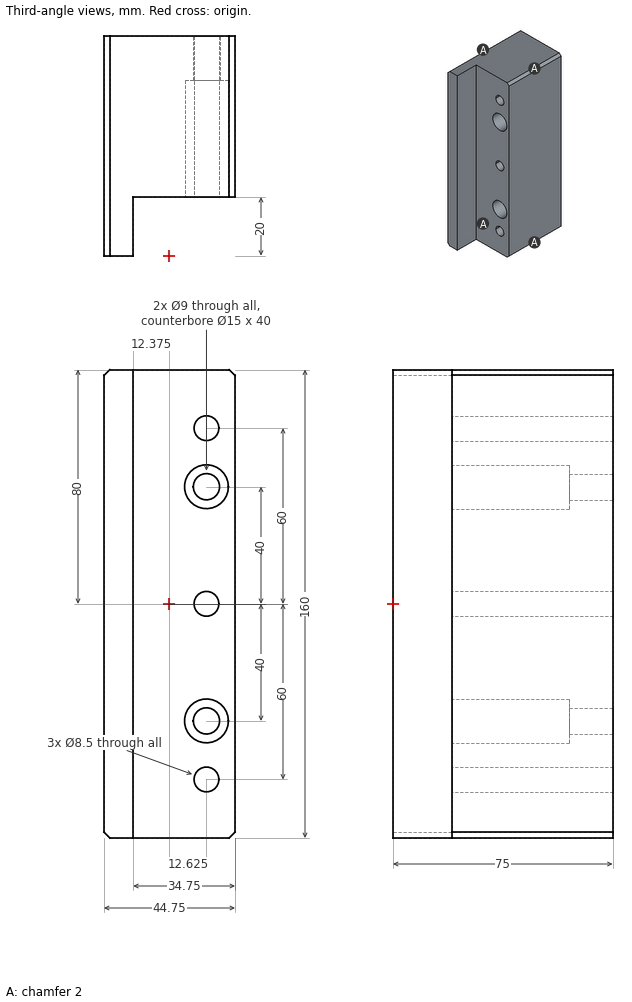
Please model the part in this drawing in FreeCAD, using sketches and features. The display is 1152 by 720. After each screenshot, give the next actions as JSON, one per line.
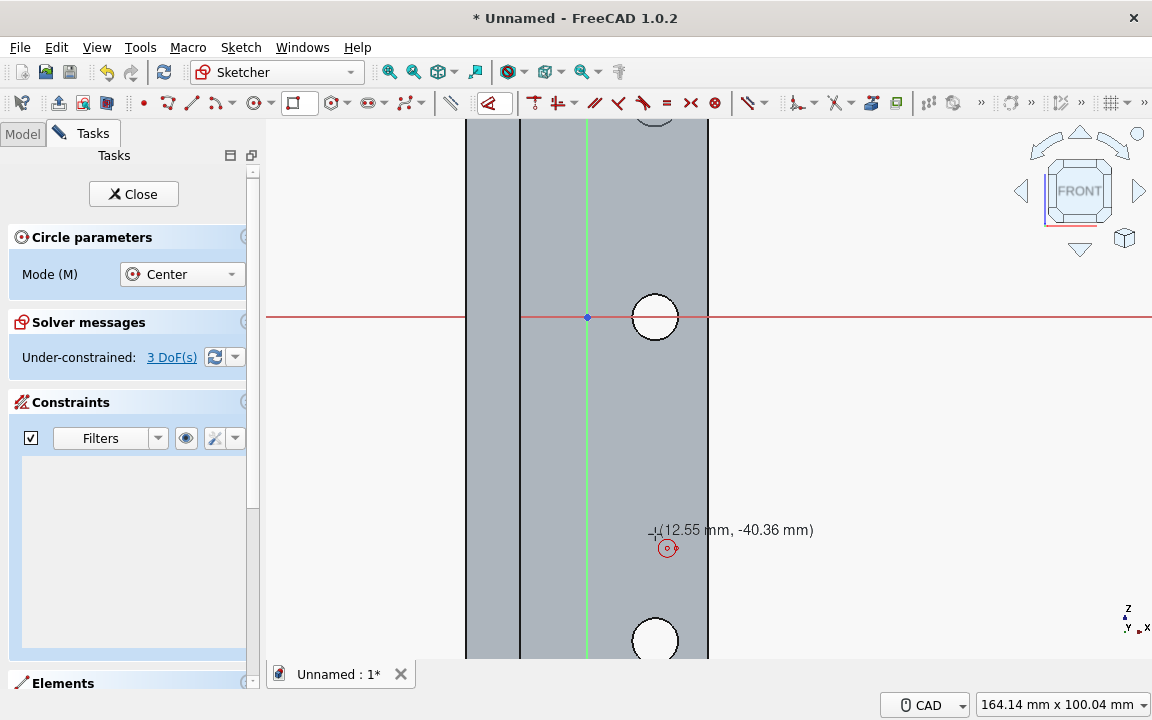
{"action": "left_click", "coordinate": [655, 533]}
{"action": "left_click", "coordinate": [672, 516]}
{"action": "key", "text": "Escape"}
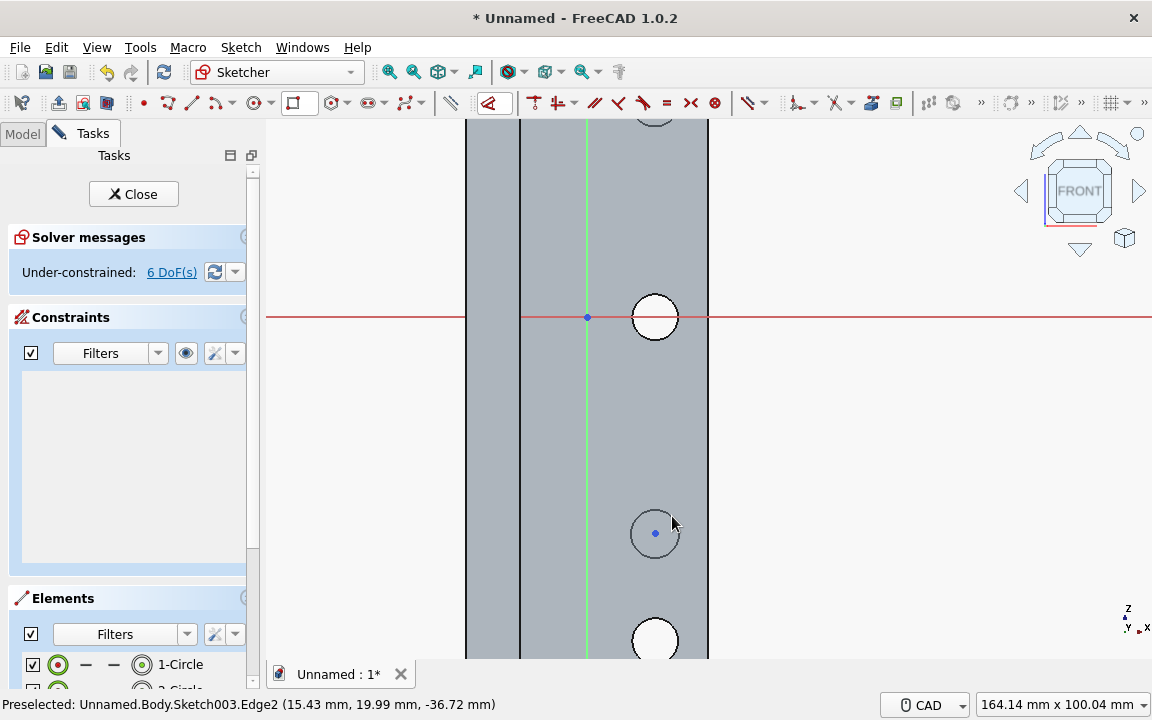
{"action": "scroll", "coordinate": [655, 535], "scroll_direction": "down", "scroll_amount": 2}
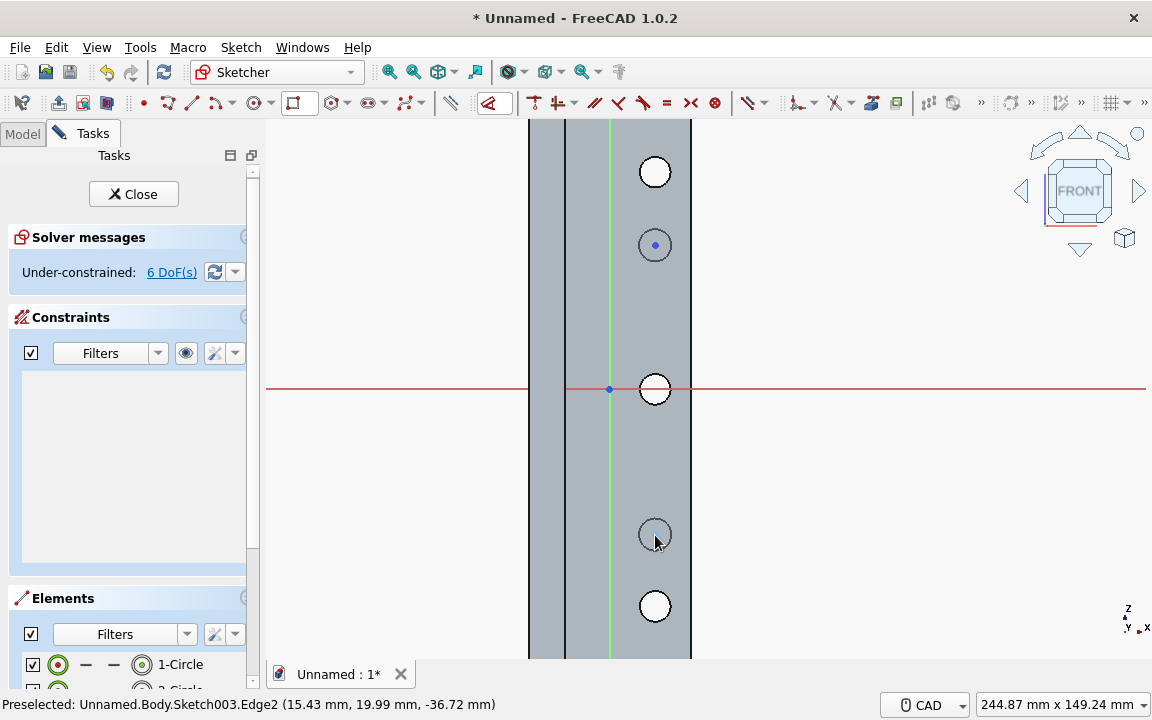
{"action": "left_click", "coordinate": [666, 234]}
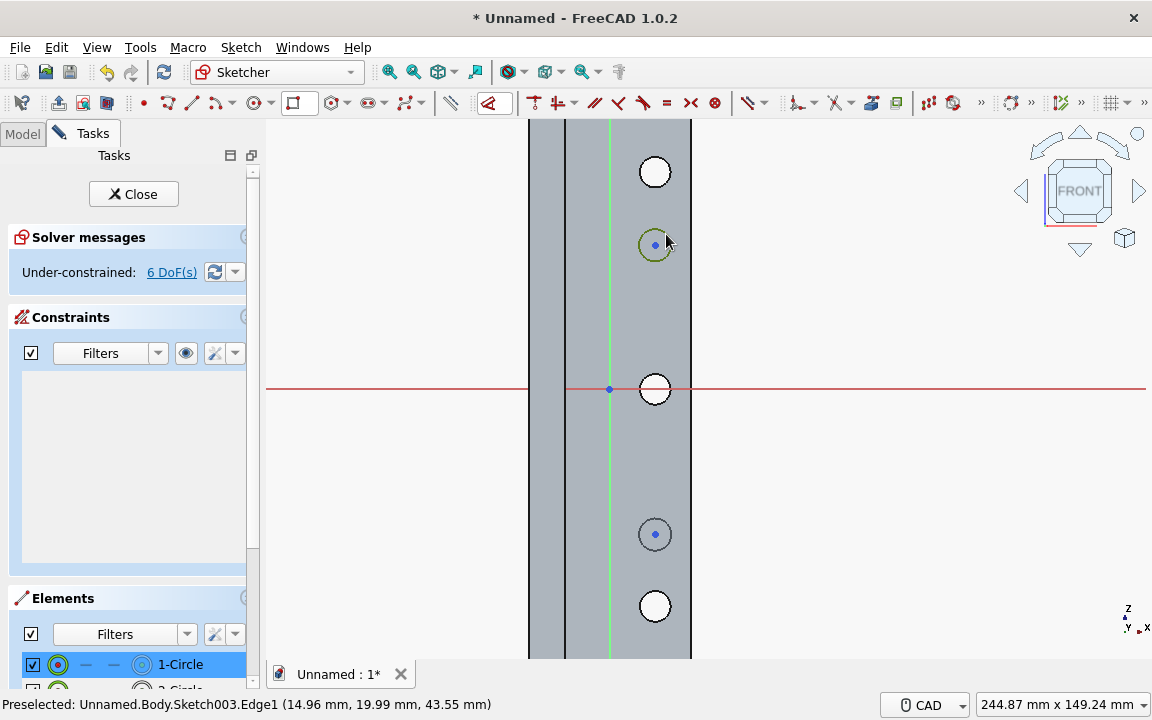
{"action": "left_click", "coordinate": [667, 523]}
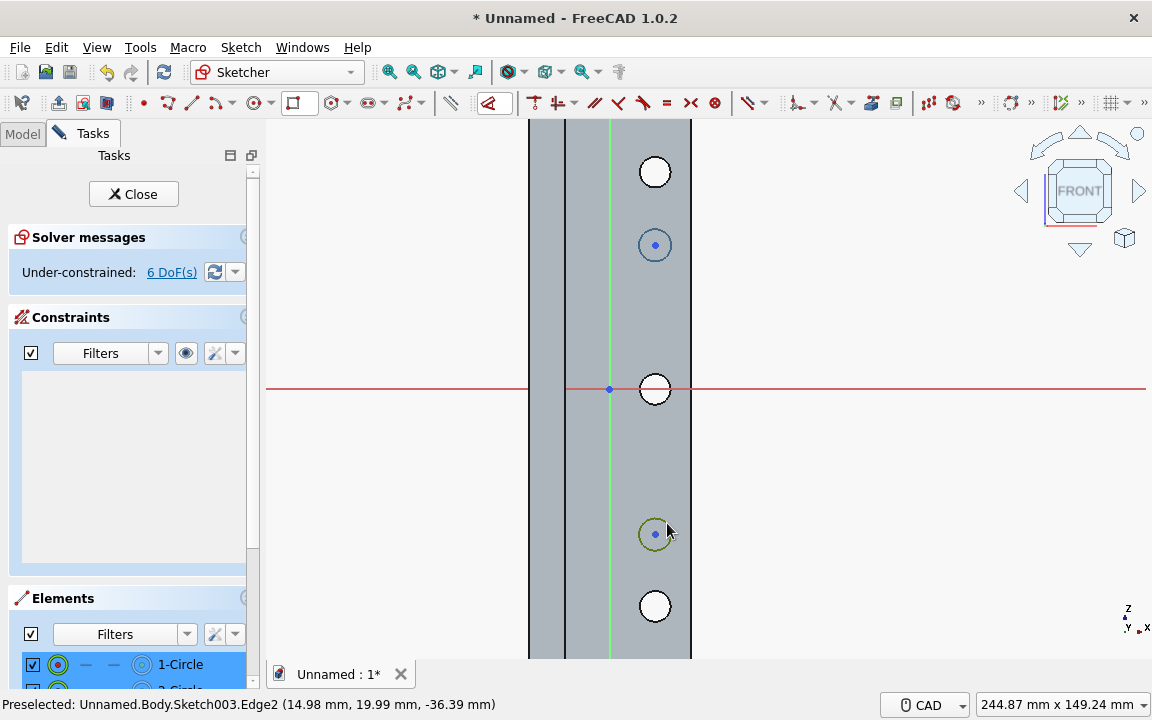
{"action": "left_click", "coordinate": [668, 104]}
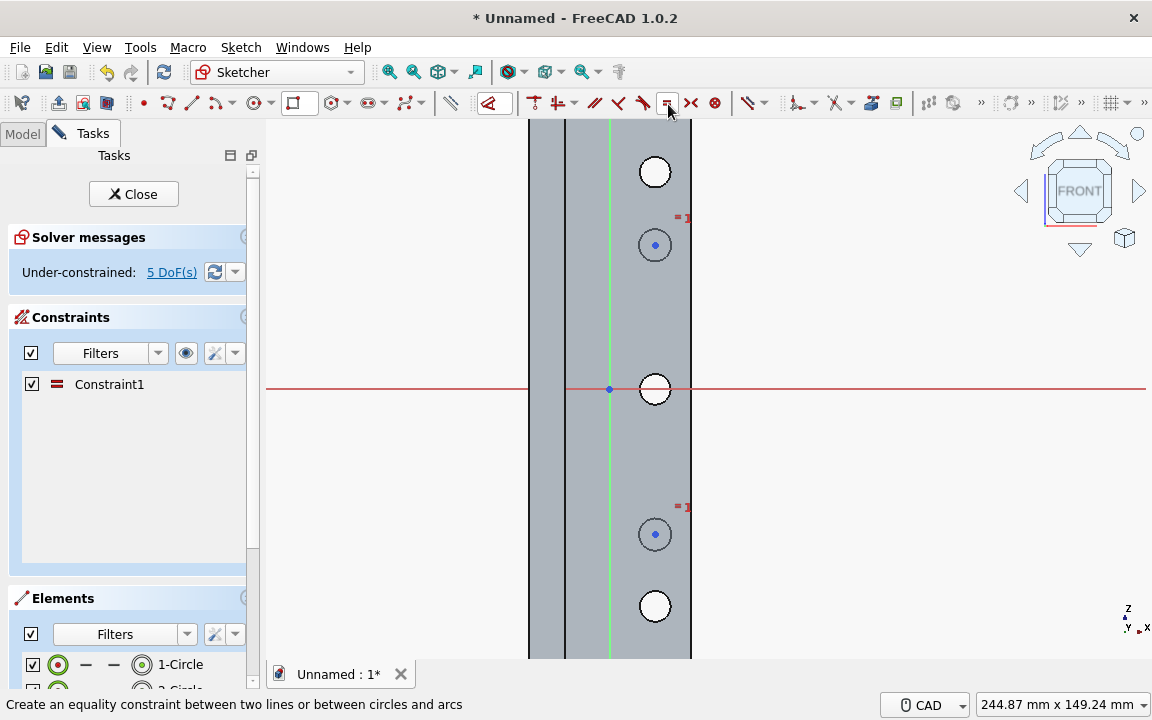
{"action": "left_click", "coordinate": [655, 245]}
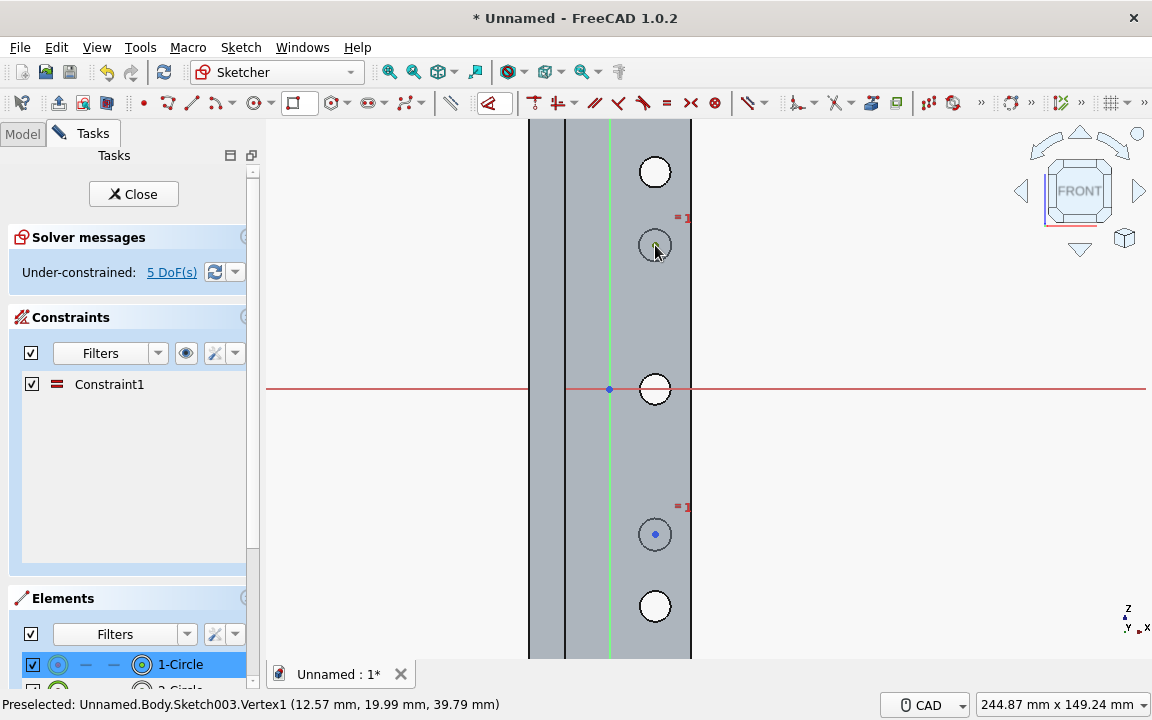
{"action": "left_click", "coordinate": [655, 535]}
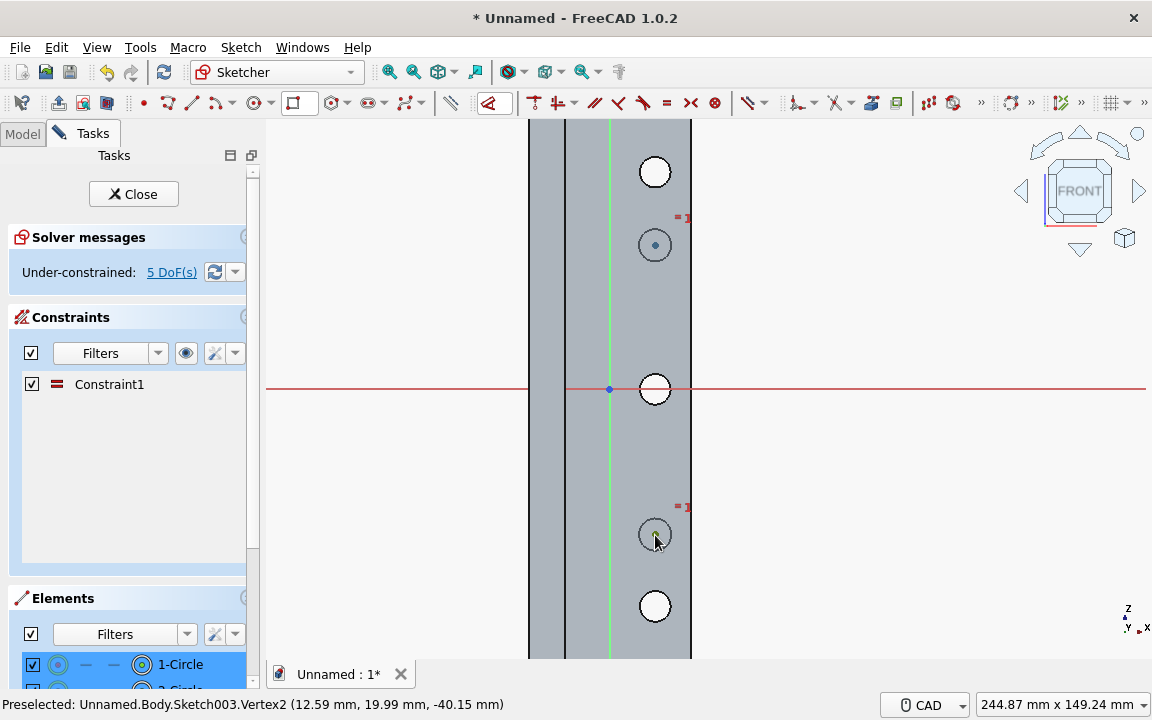
{"action": "key", "text": "v"}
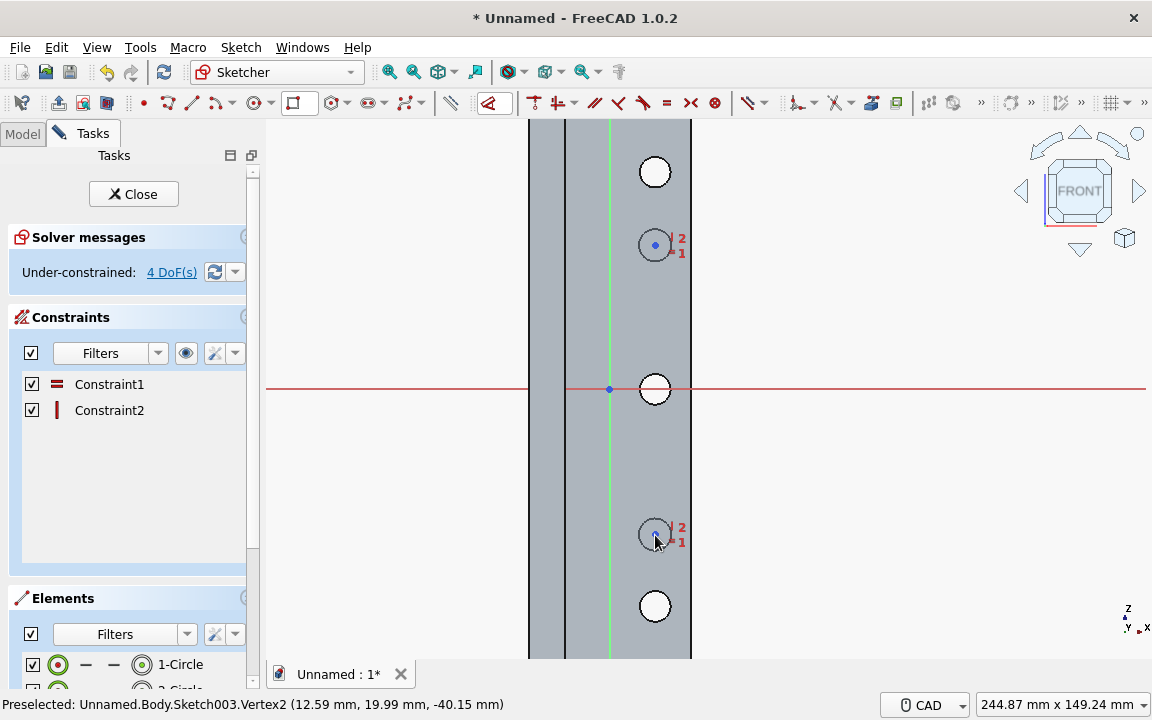
{"action": "left_click", "coordinate": [488, 104]}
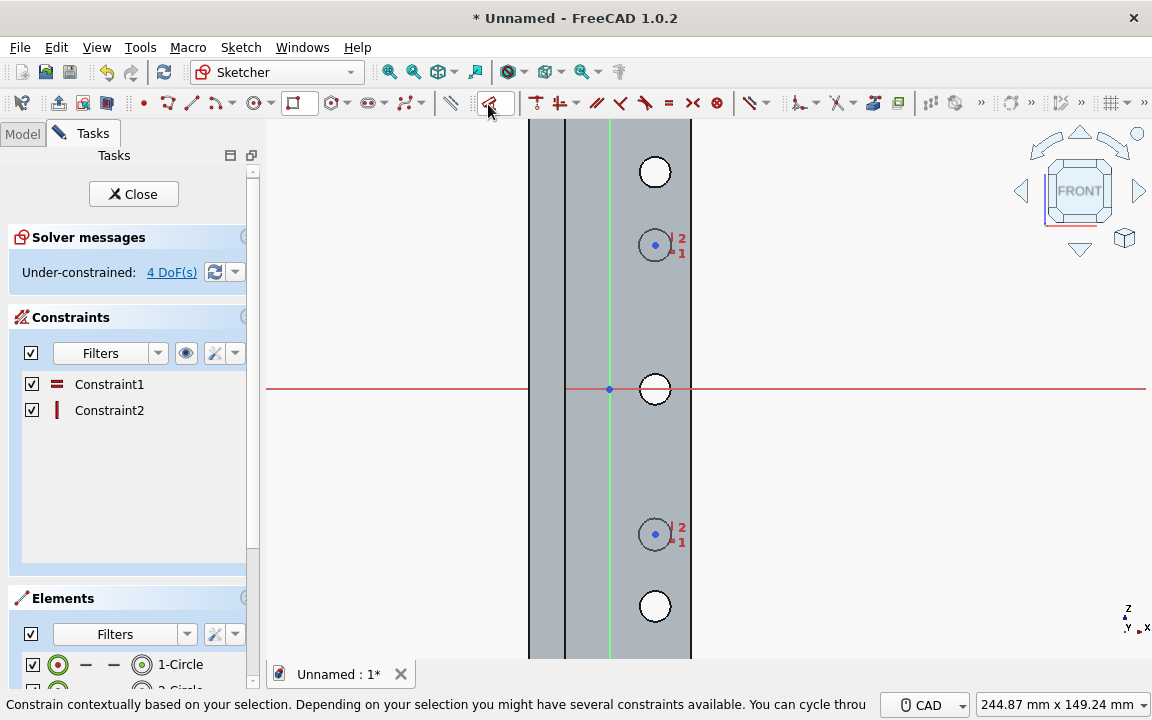
{"action": "left_click", "coordinate": [666, 234]}
{"action": "left_click", "coordinate": [688, 211]}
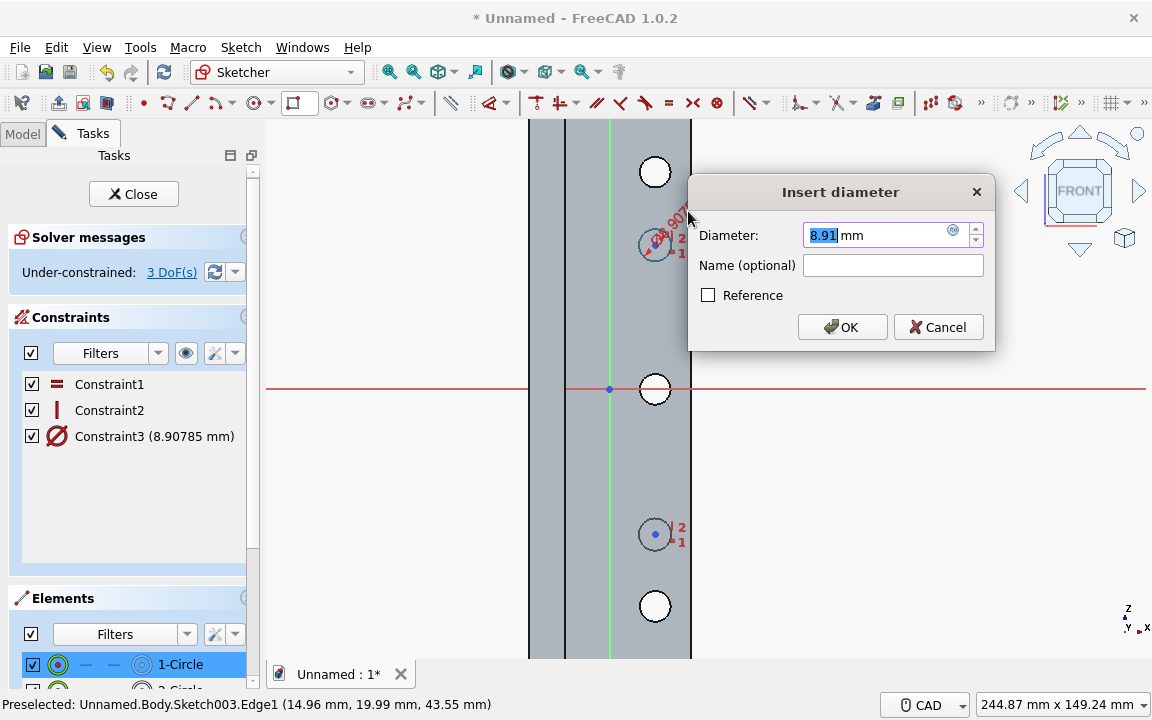
{"action": "type", "text": "9"}
{"action": "key", "text": "Return"}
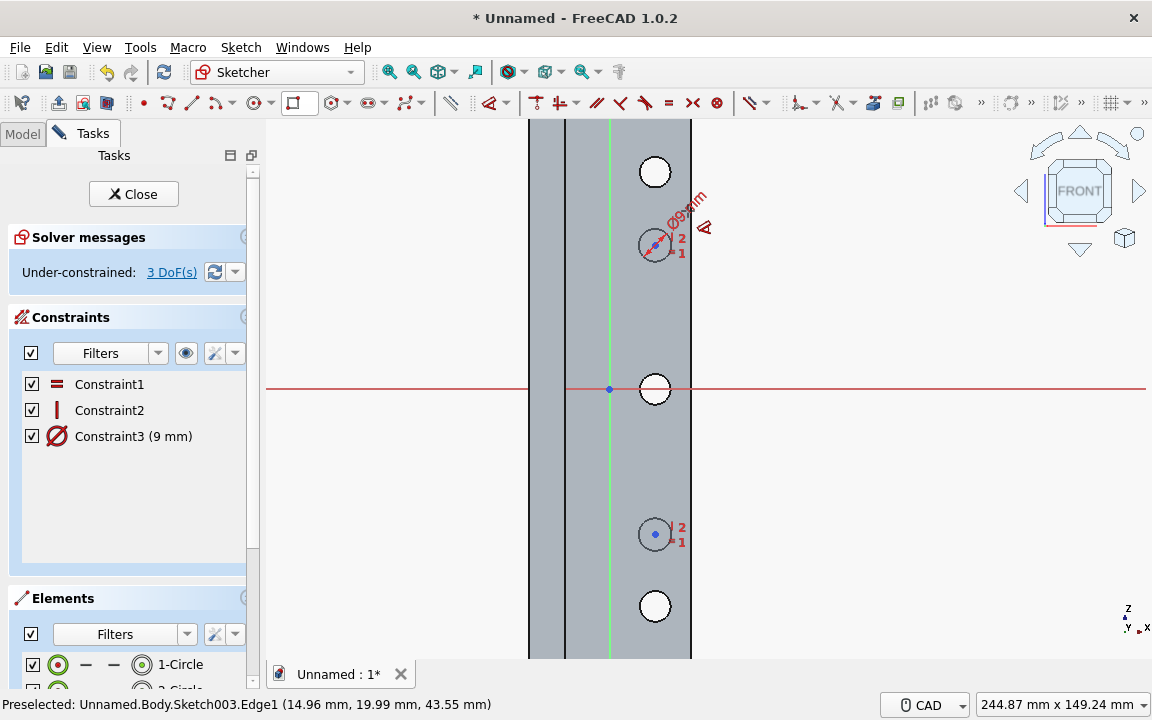
{"action": "left_click", "coordinate": [655, 245]}
{"action": "left_click", "coordinate": [576, 317]}